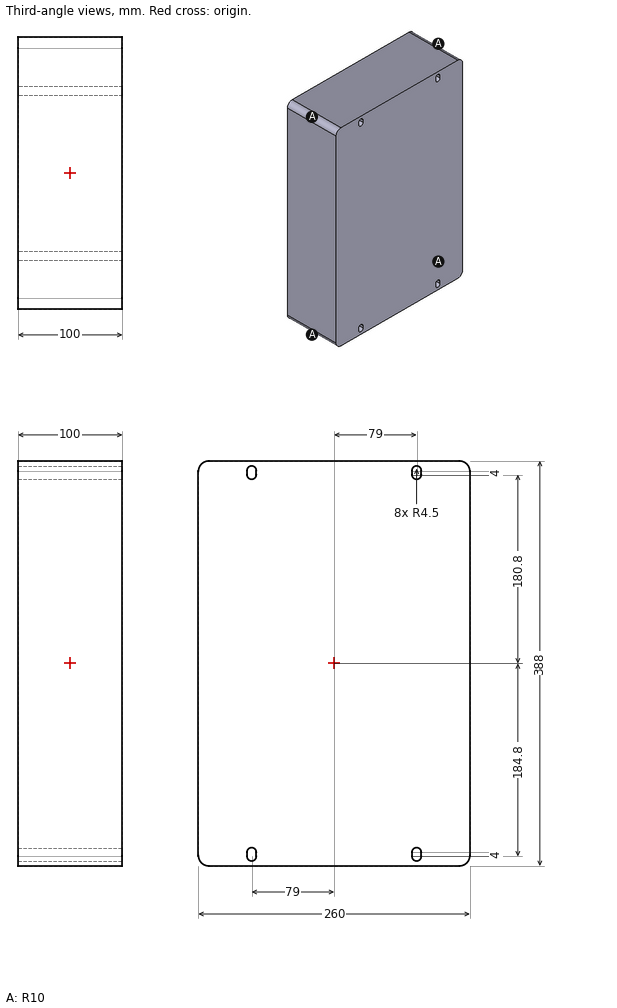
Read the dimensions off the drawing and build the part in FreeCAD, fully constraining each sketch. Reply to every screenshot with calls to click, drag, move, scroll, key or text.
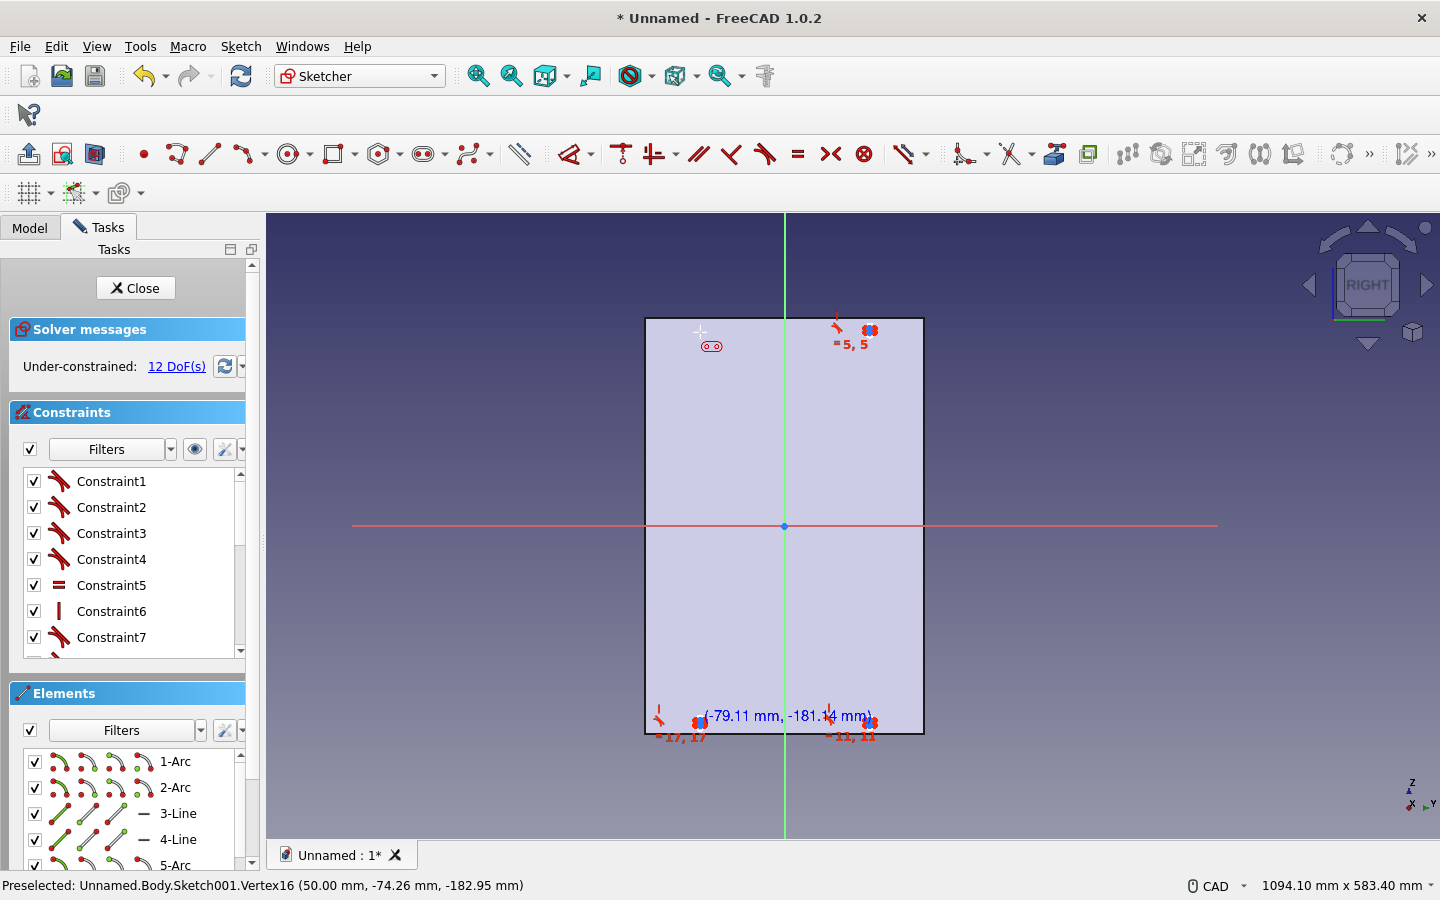
click(700, 332)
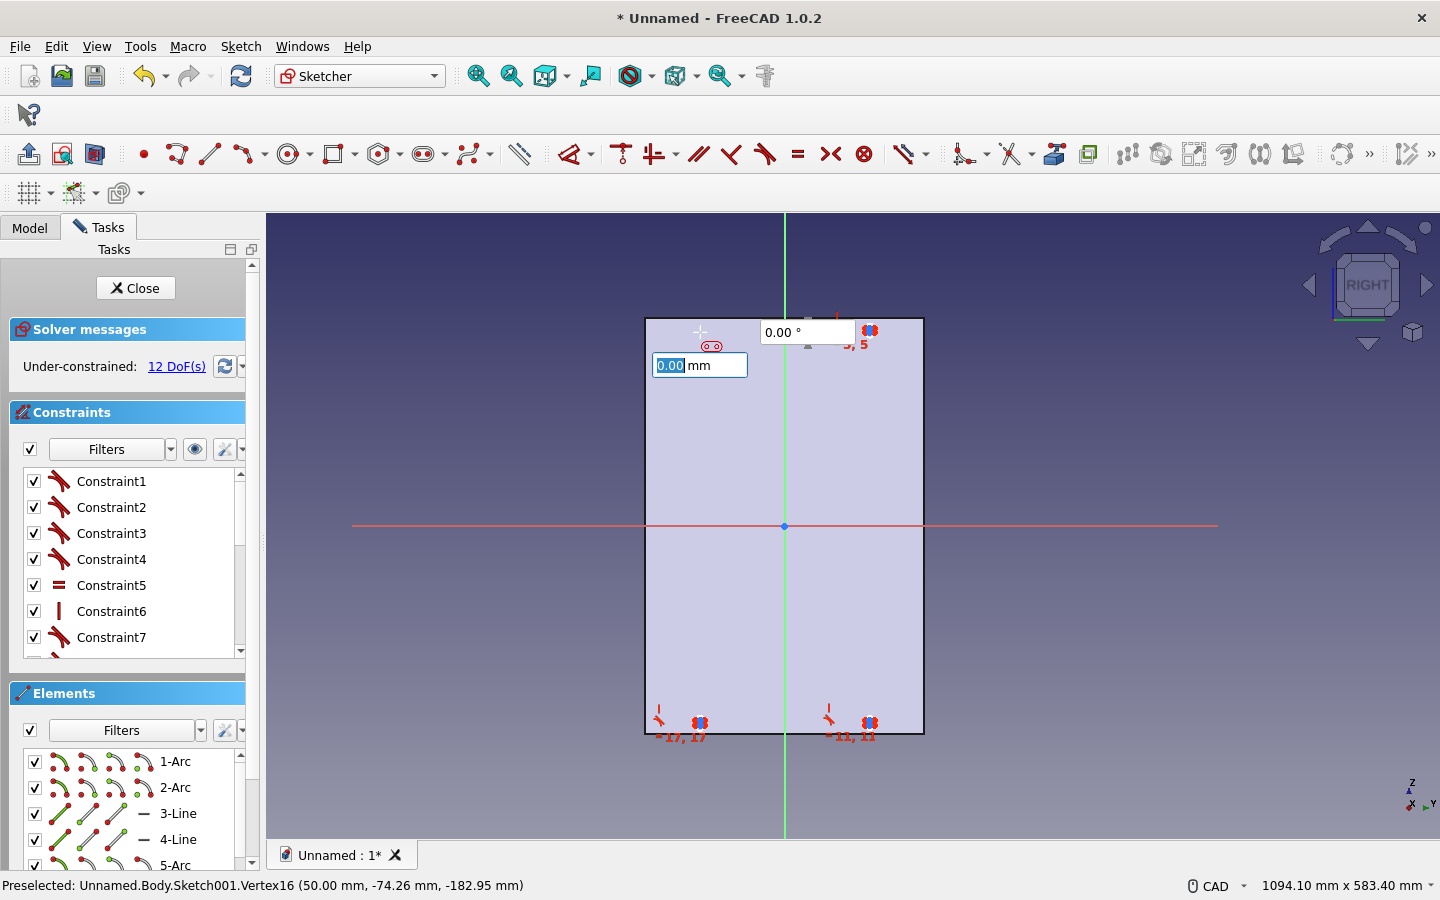
scroll(700, 328, up, 7)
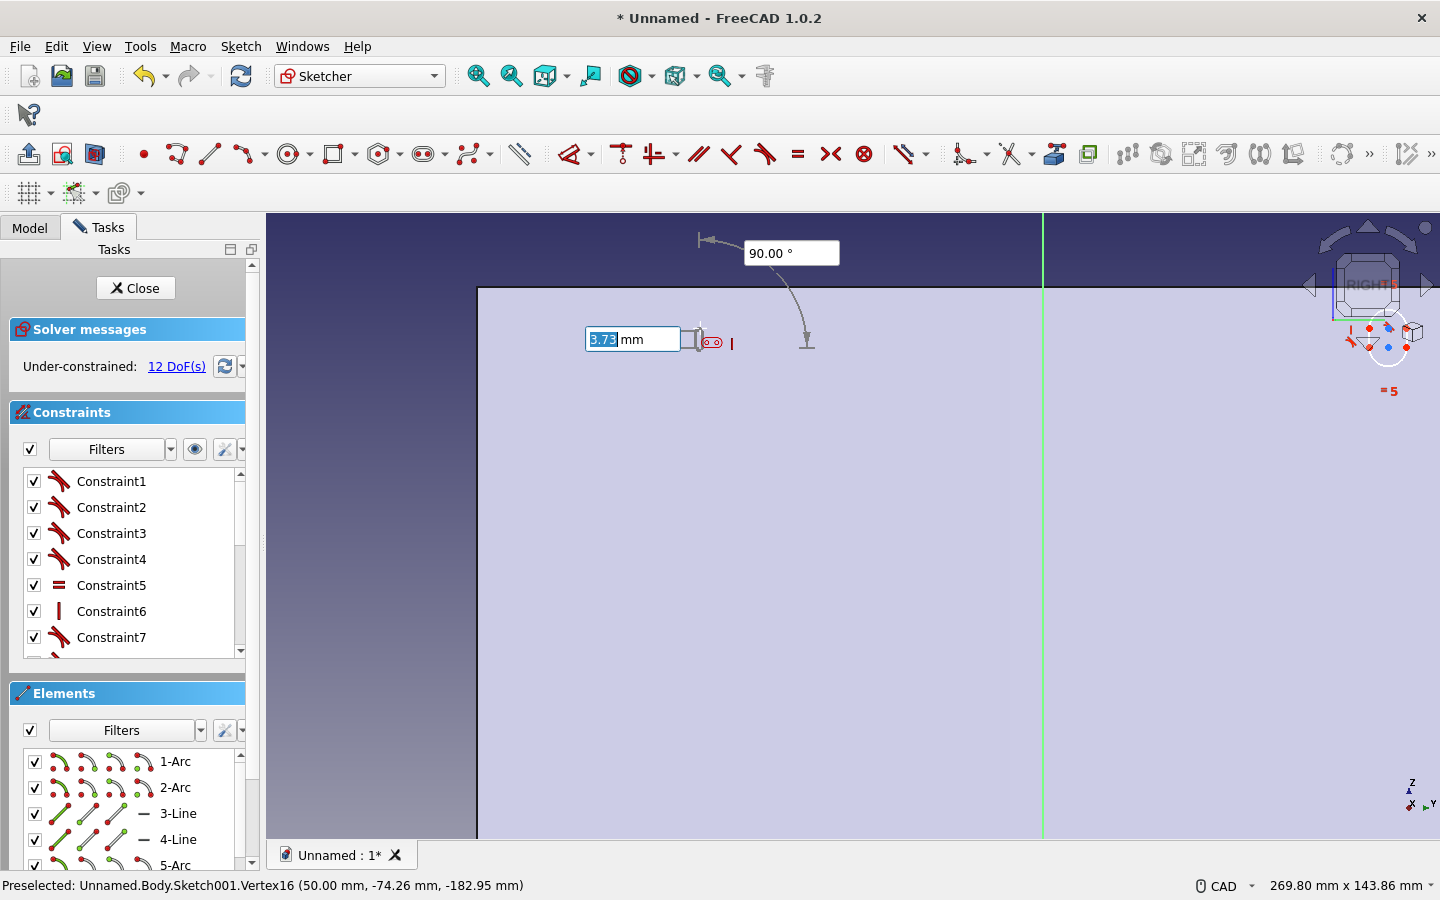
click(699, 327)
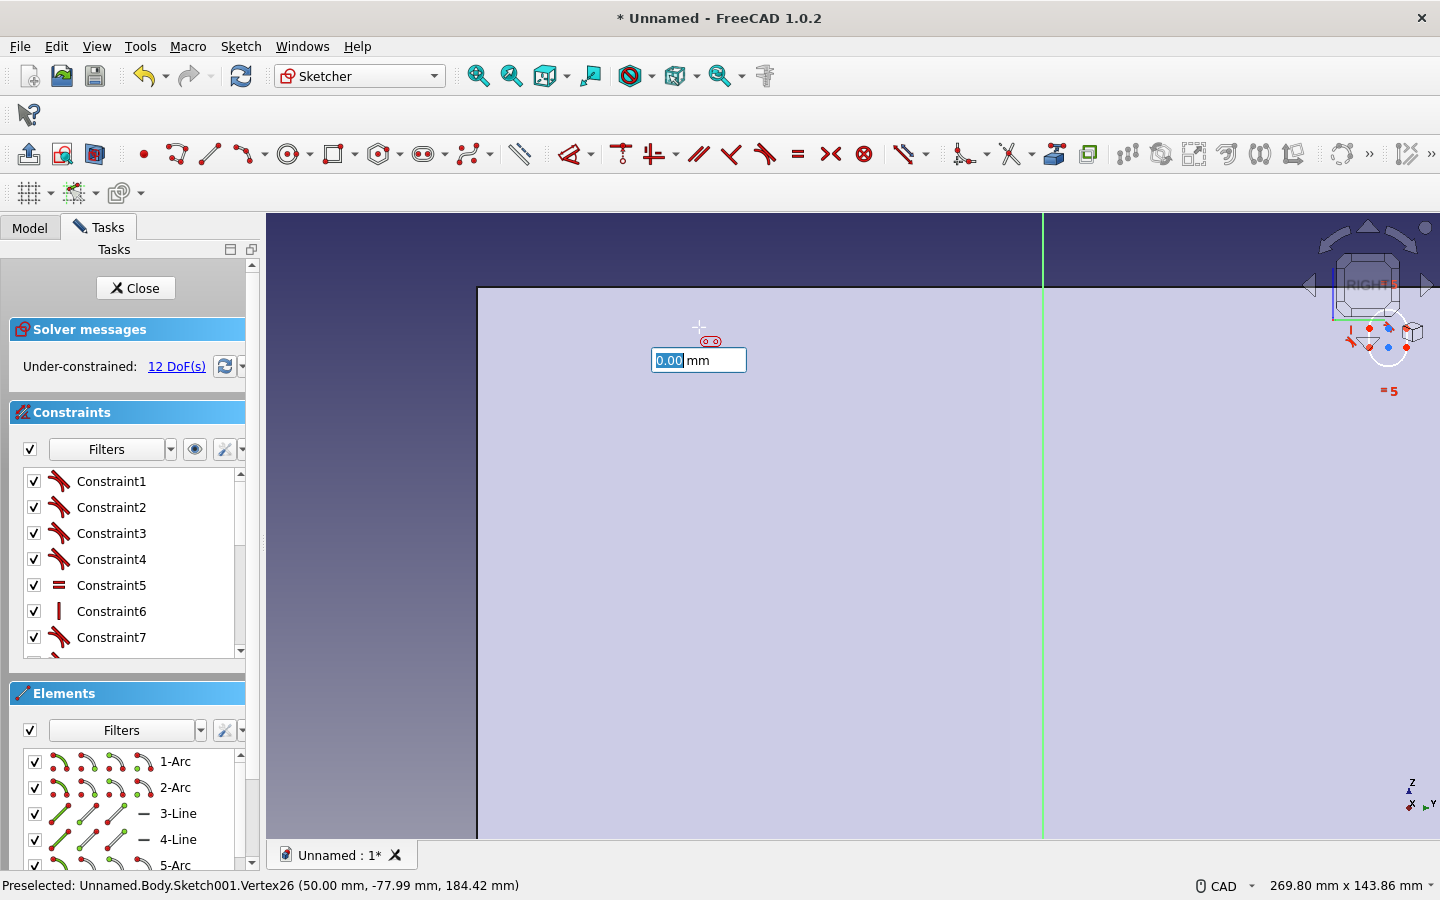
click(719, 336)
key(Escape)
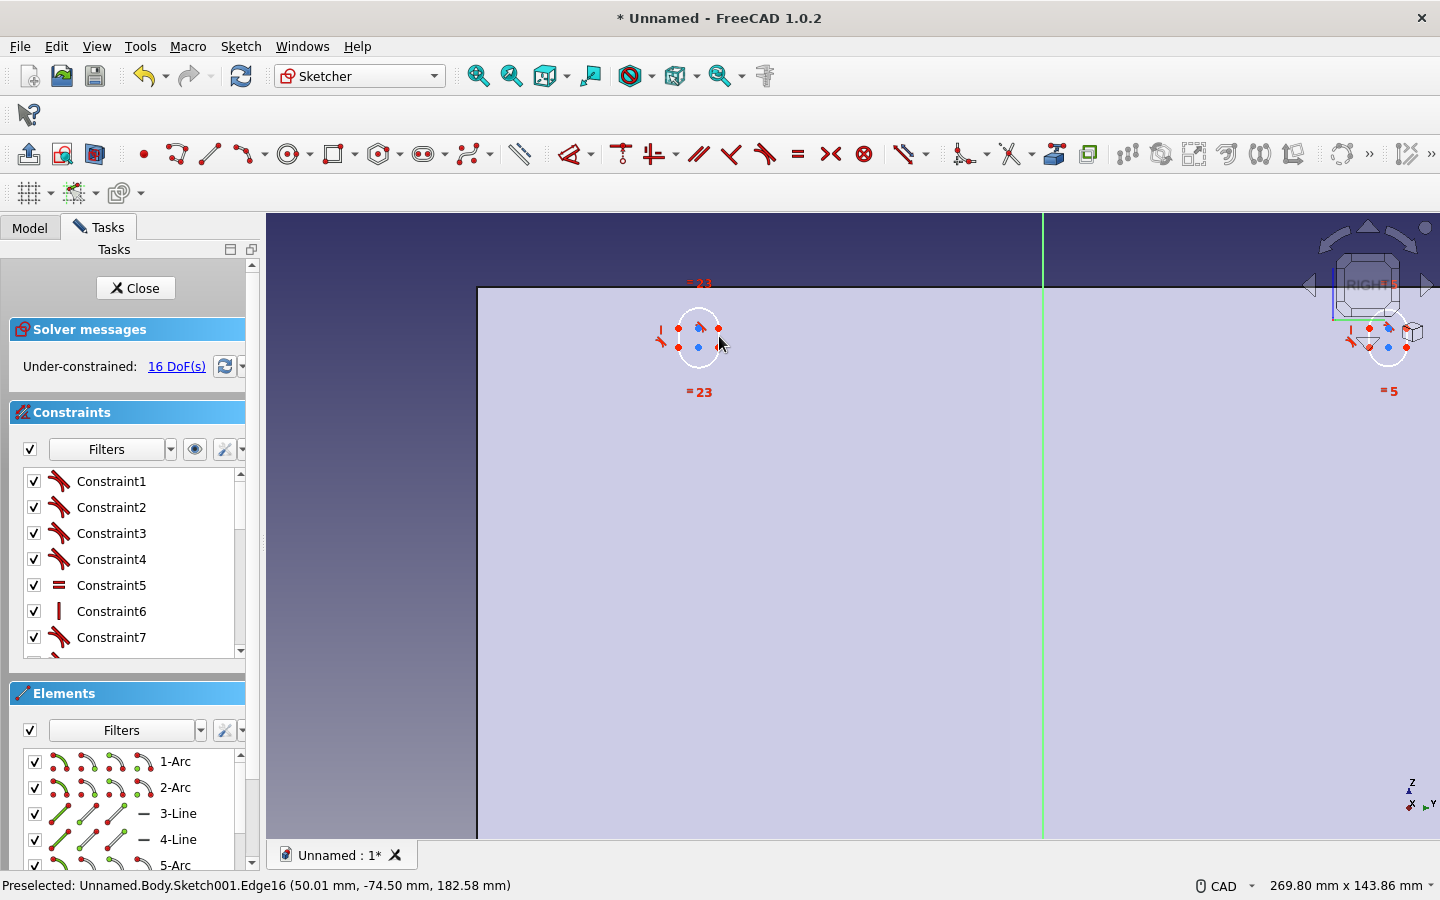
scroll(700, 328, down, 7)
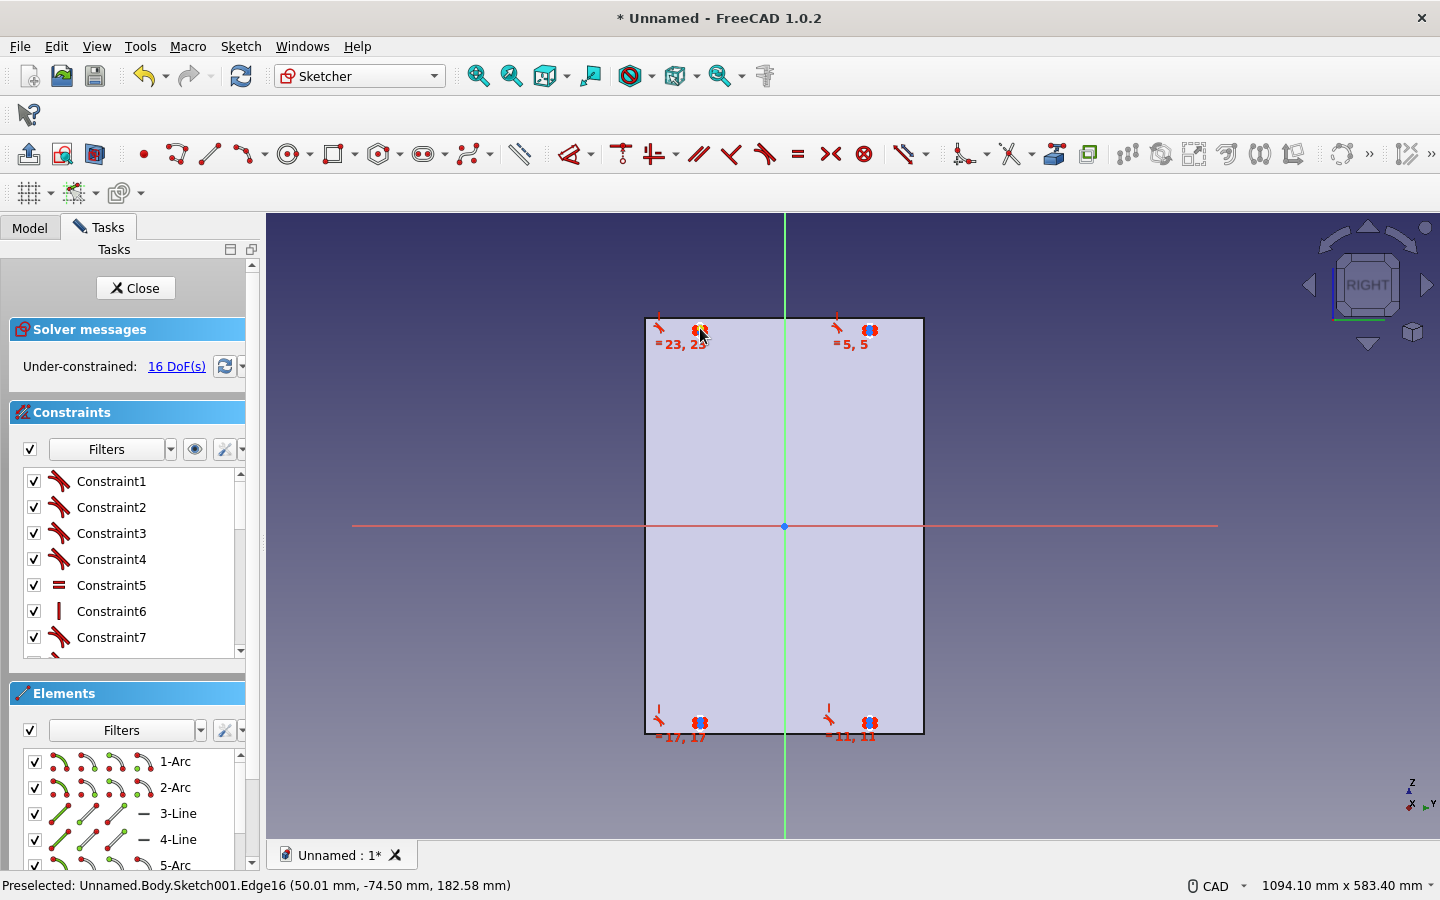
scroll(867, 337, up, 6)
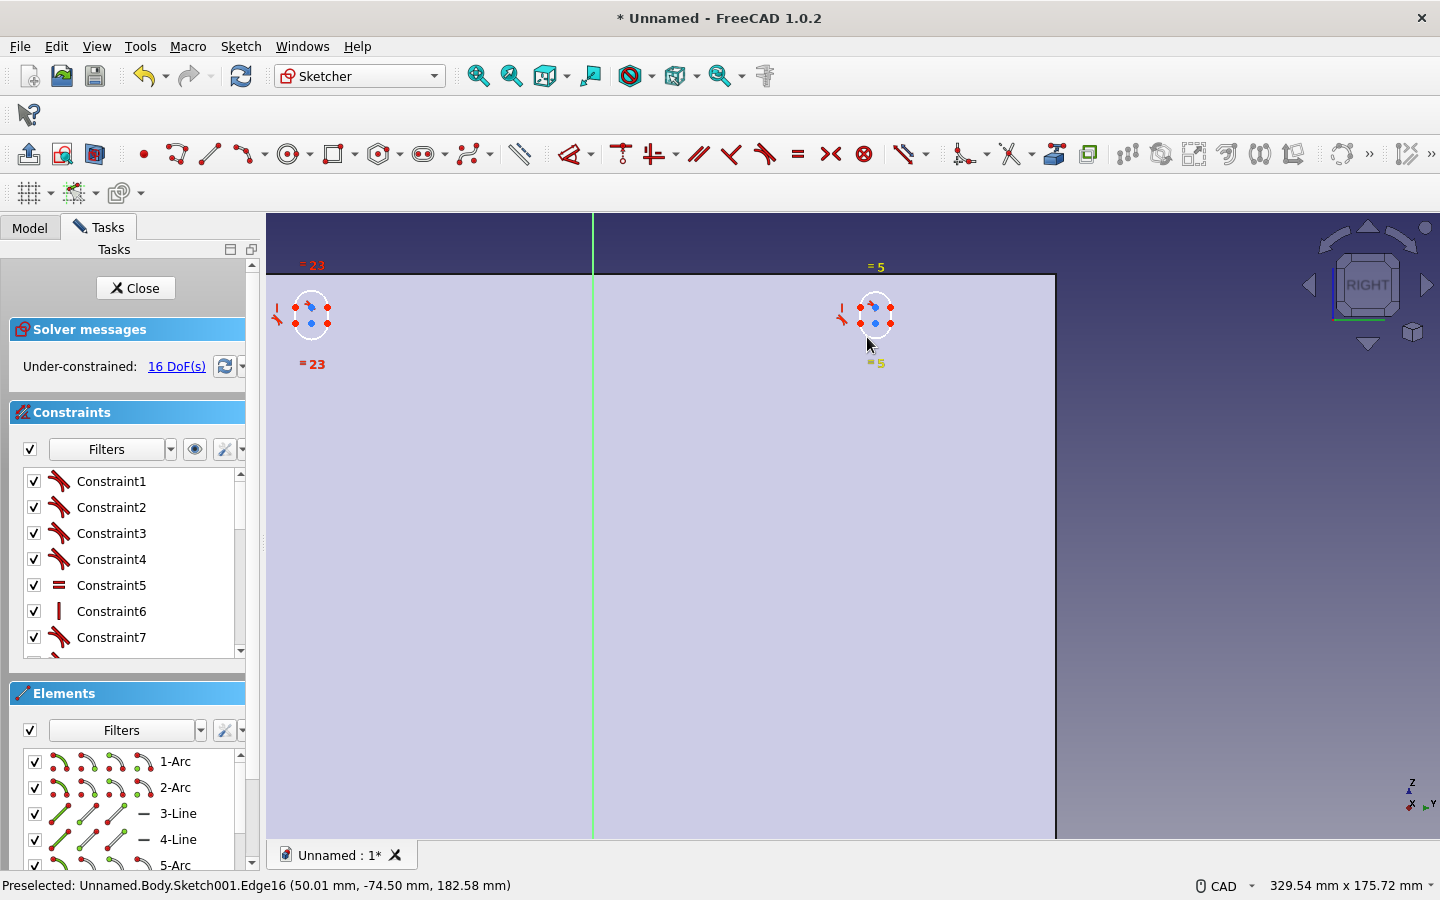
click(867, 335)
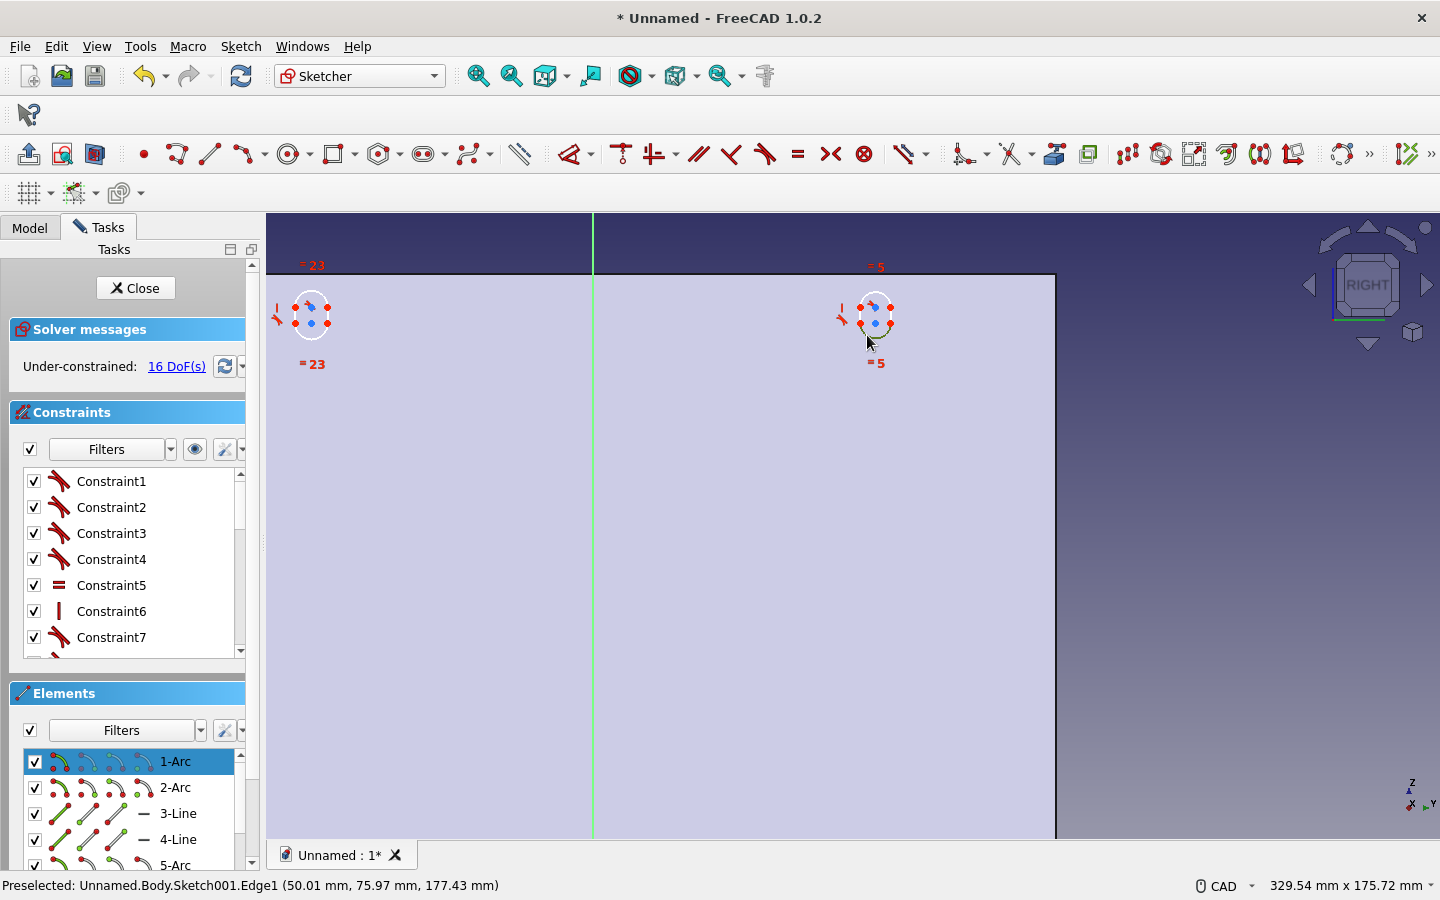
scroll(867, 337, down, 6)